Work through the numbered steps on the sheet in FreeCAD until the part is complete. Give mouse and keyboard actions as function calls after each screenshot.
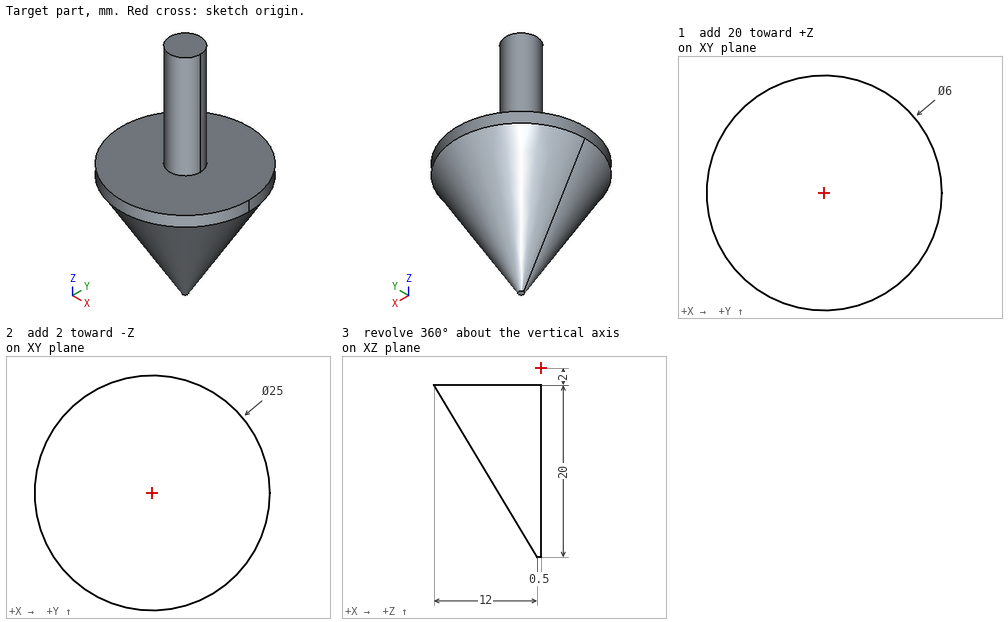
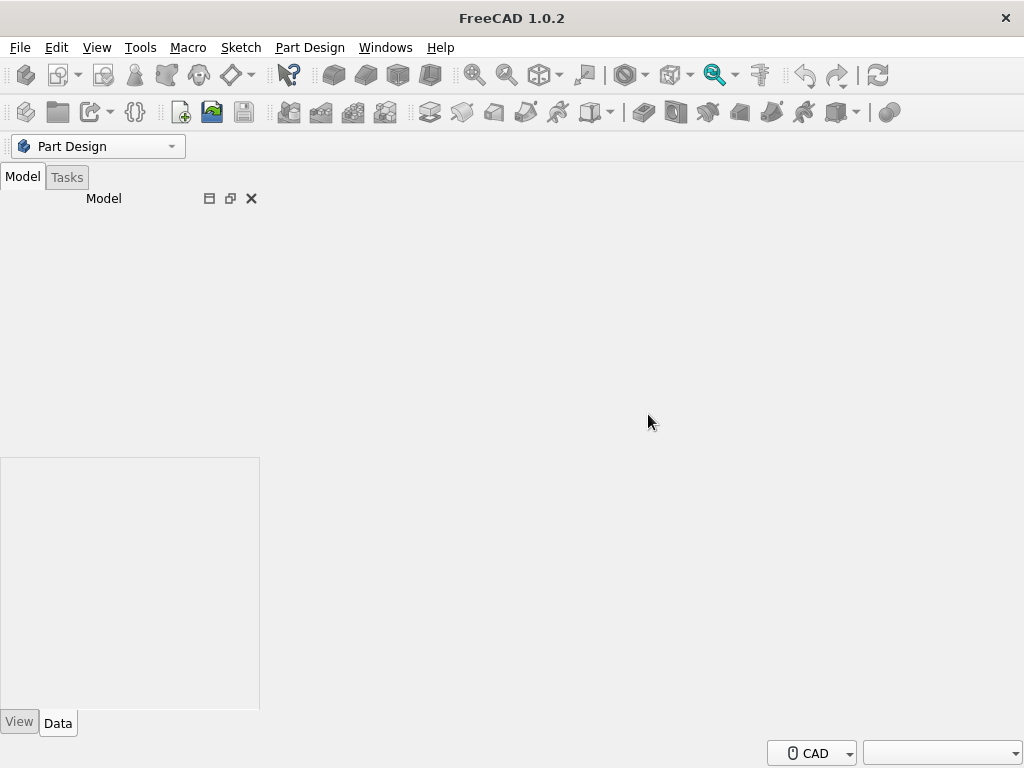
click(180, 112)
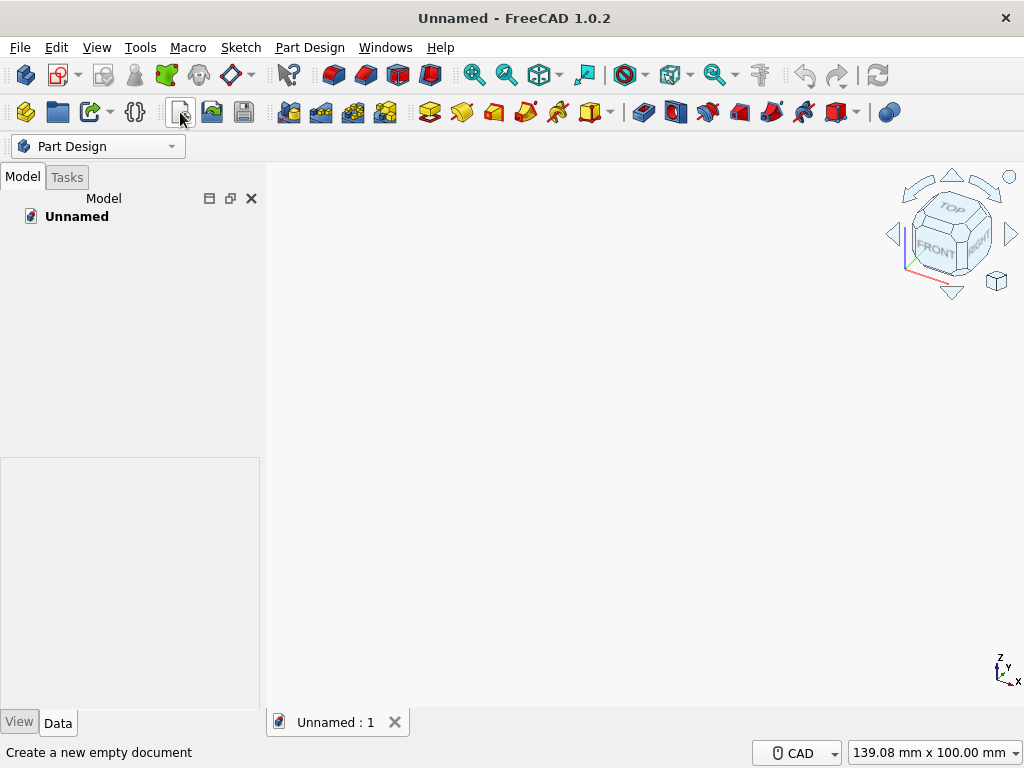
click(58, 76)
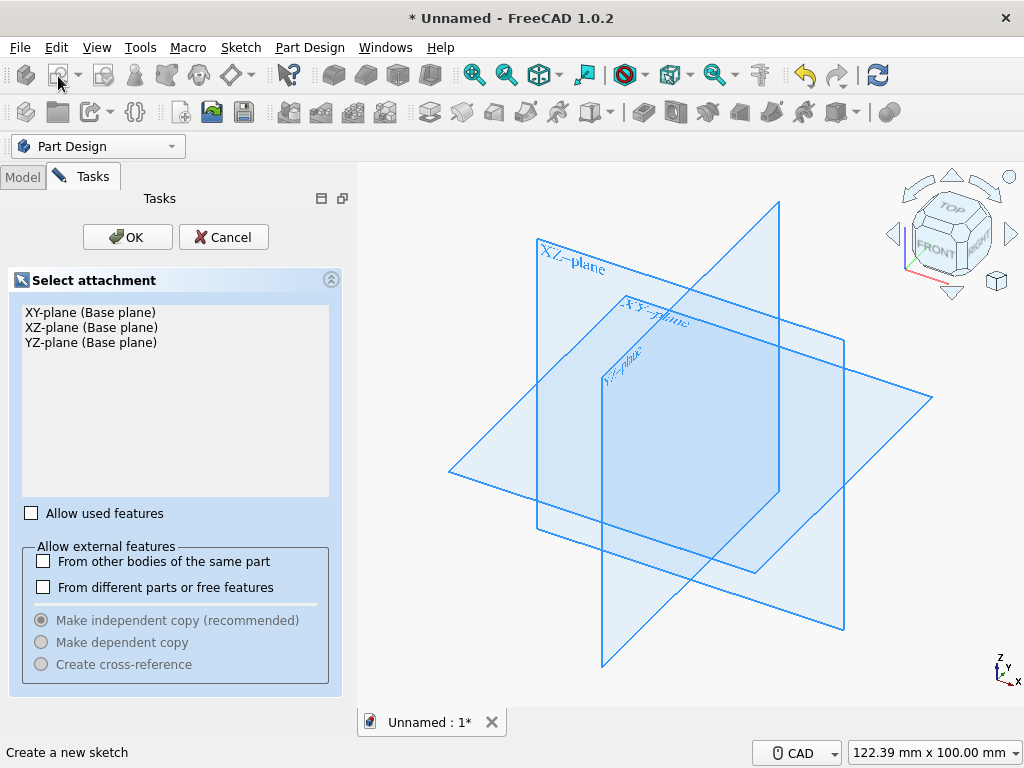
click(82, 312)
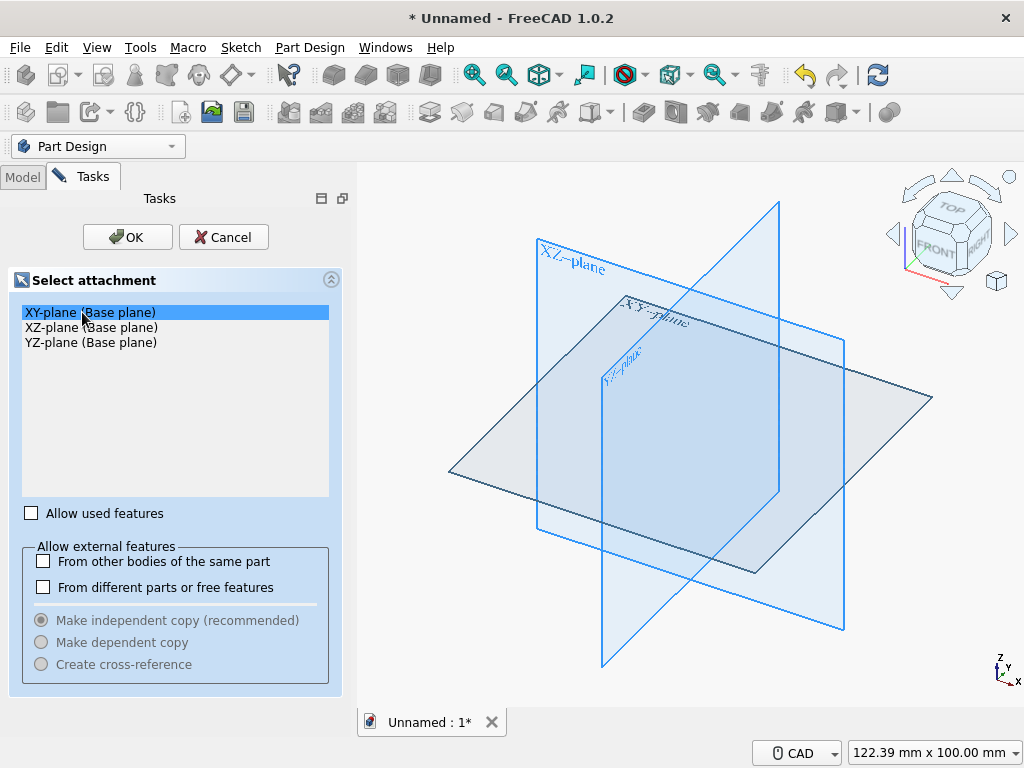
click(128, 237)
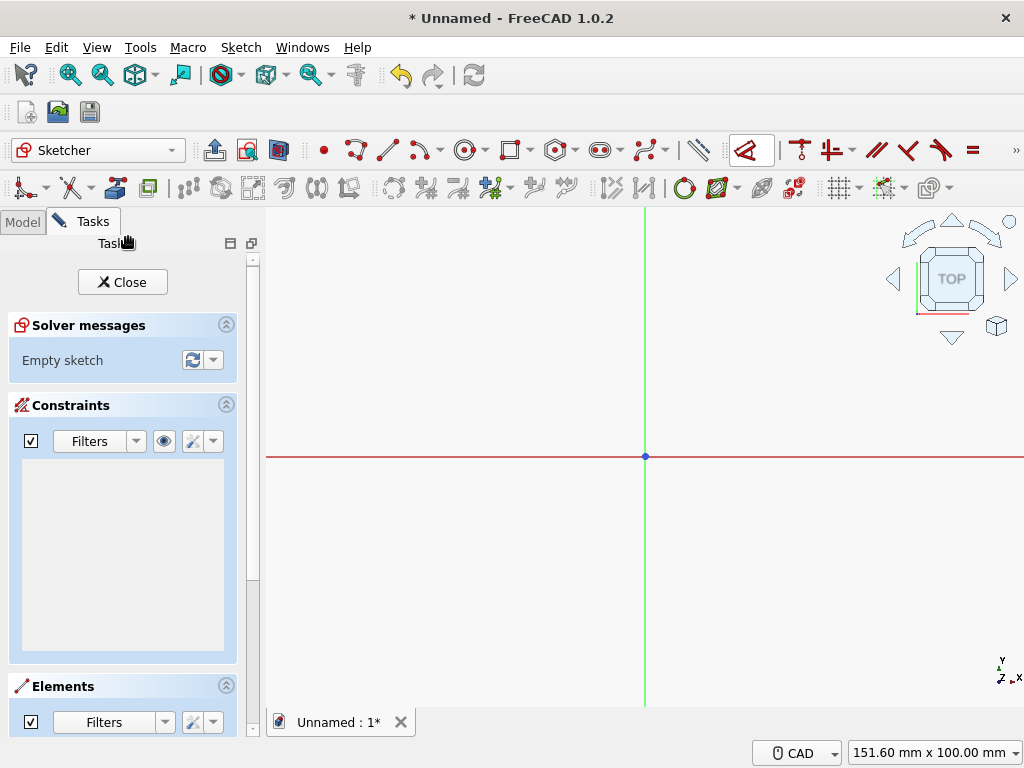
scroll(652, 457, up, 12)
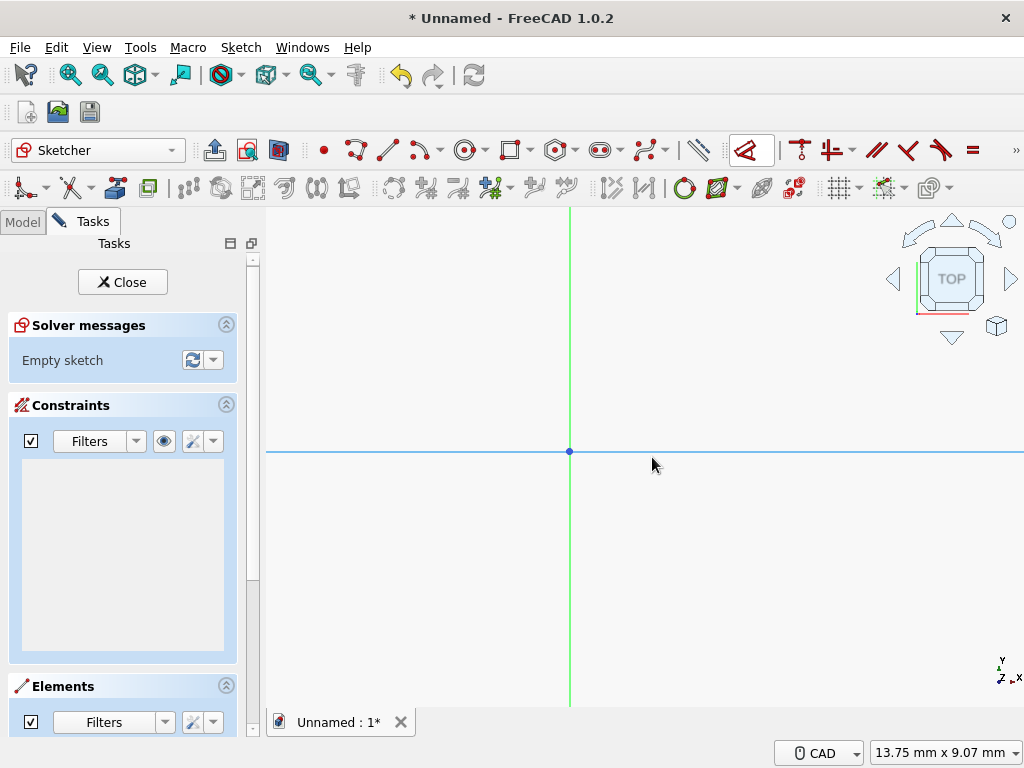
click(466, 150)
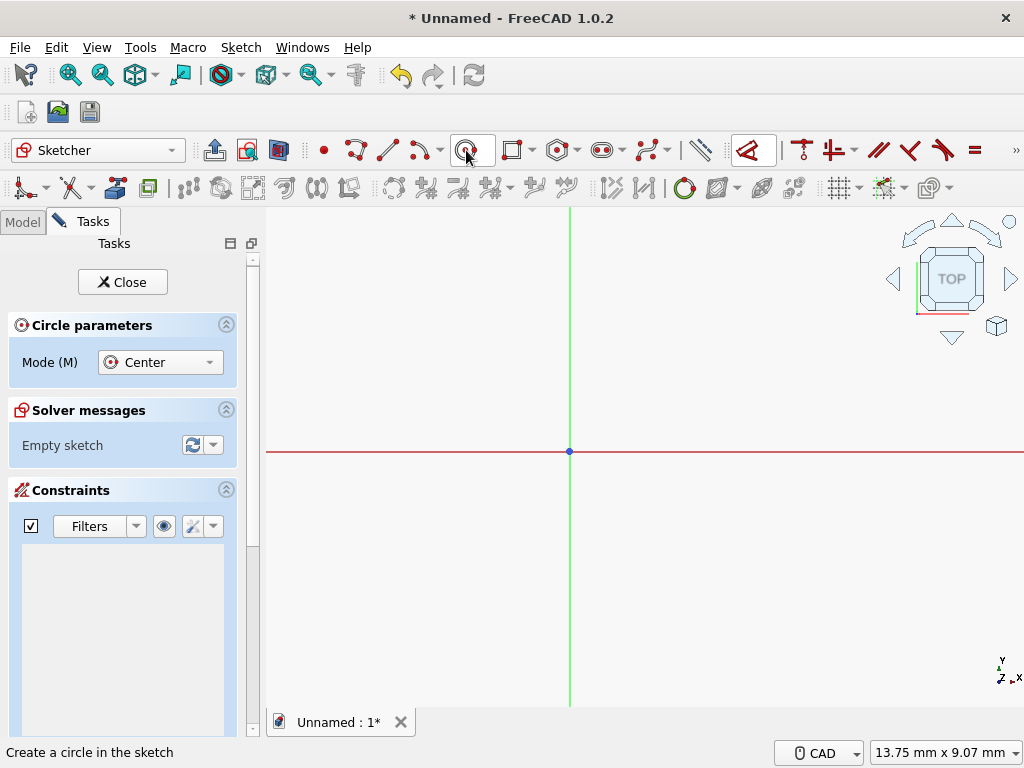
click(570, 452)
click(687, 335)
key(Escape)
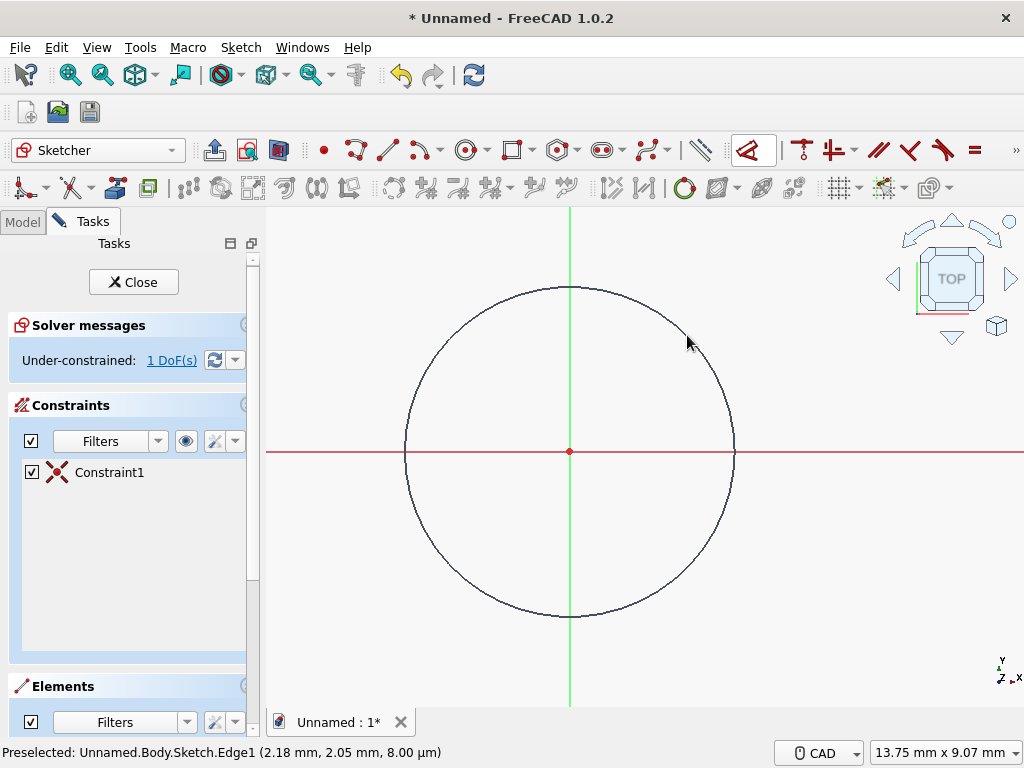
click(748, 150)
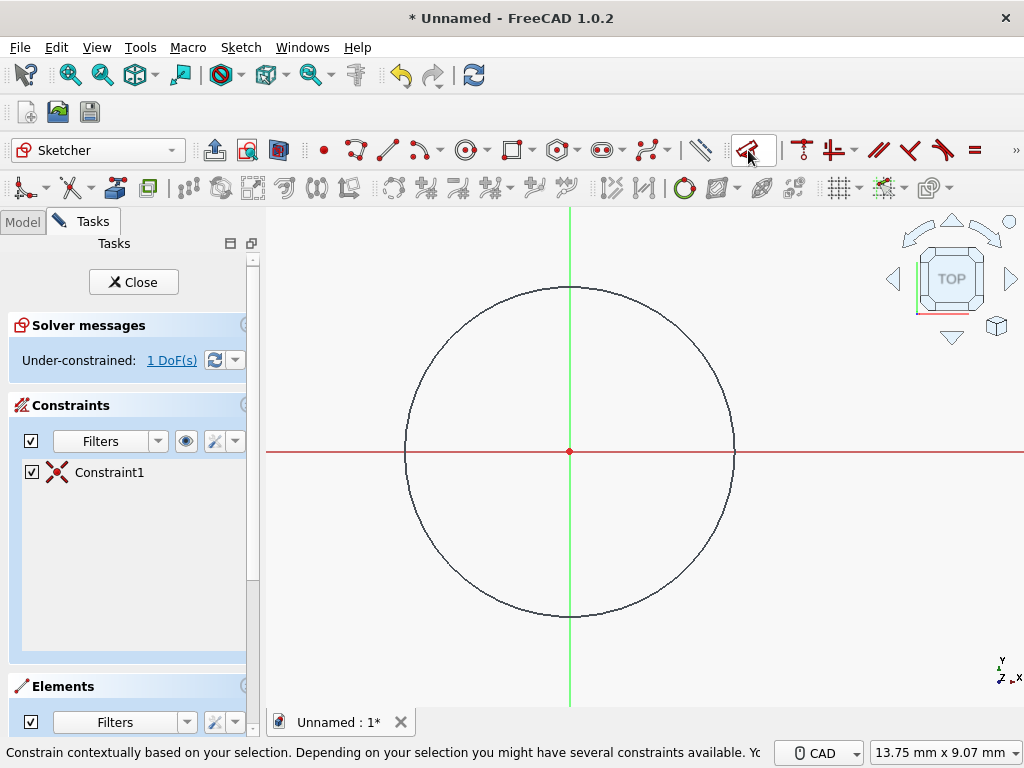
click(686, 335)
click(709, 312)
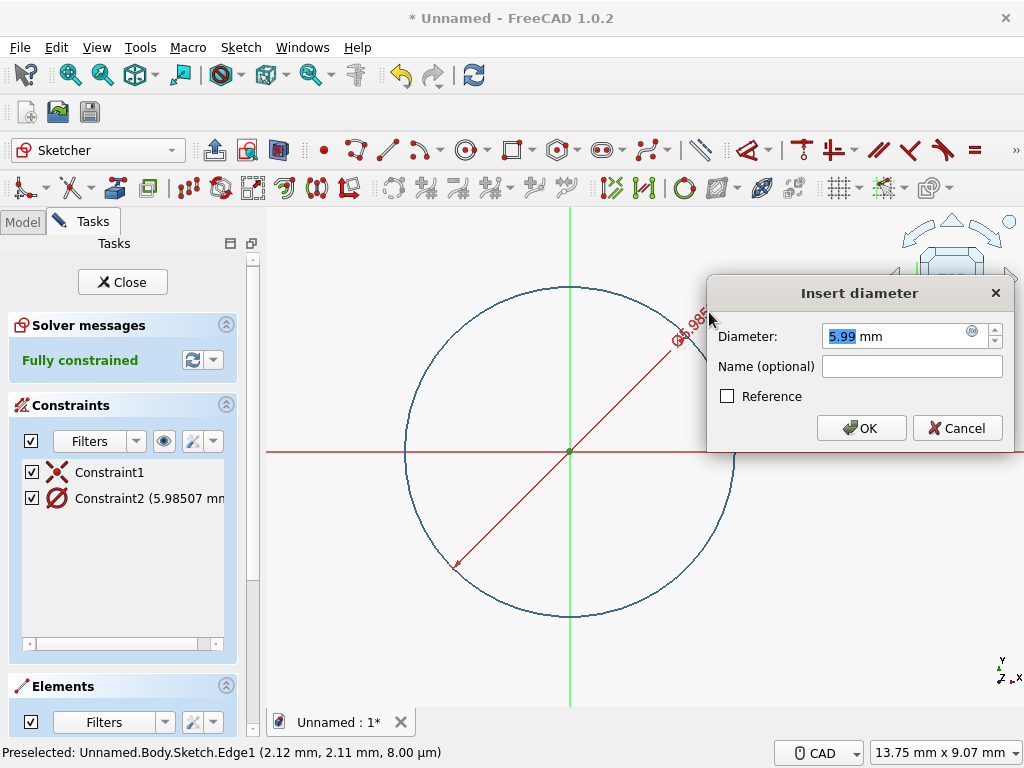
text(6)
key(Return)
key(Escape)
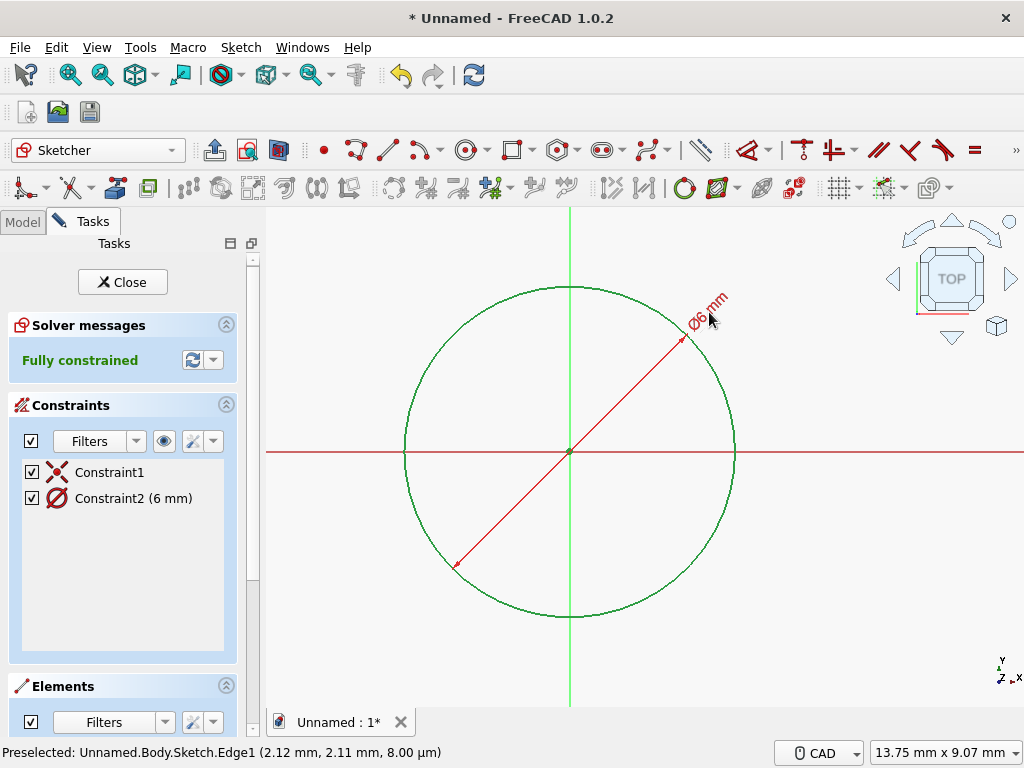
click(123, 282)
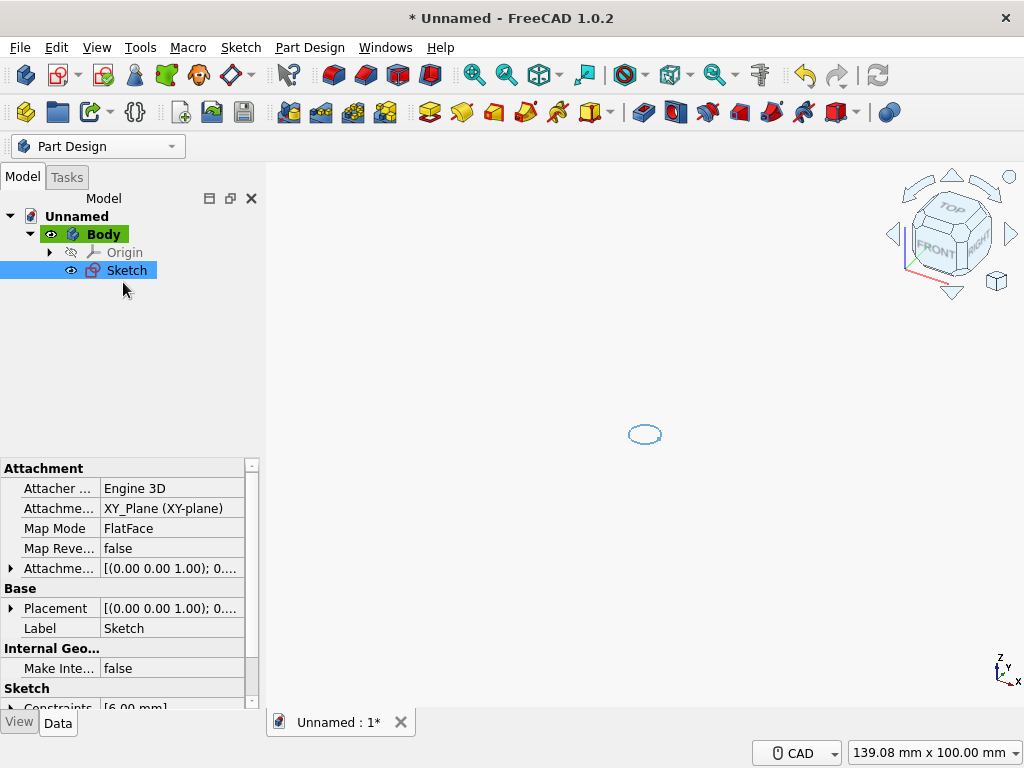
click(430, 112)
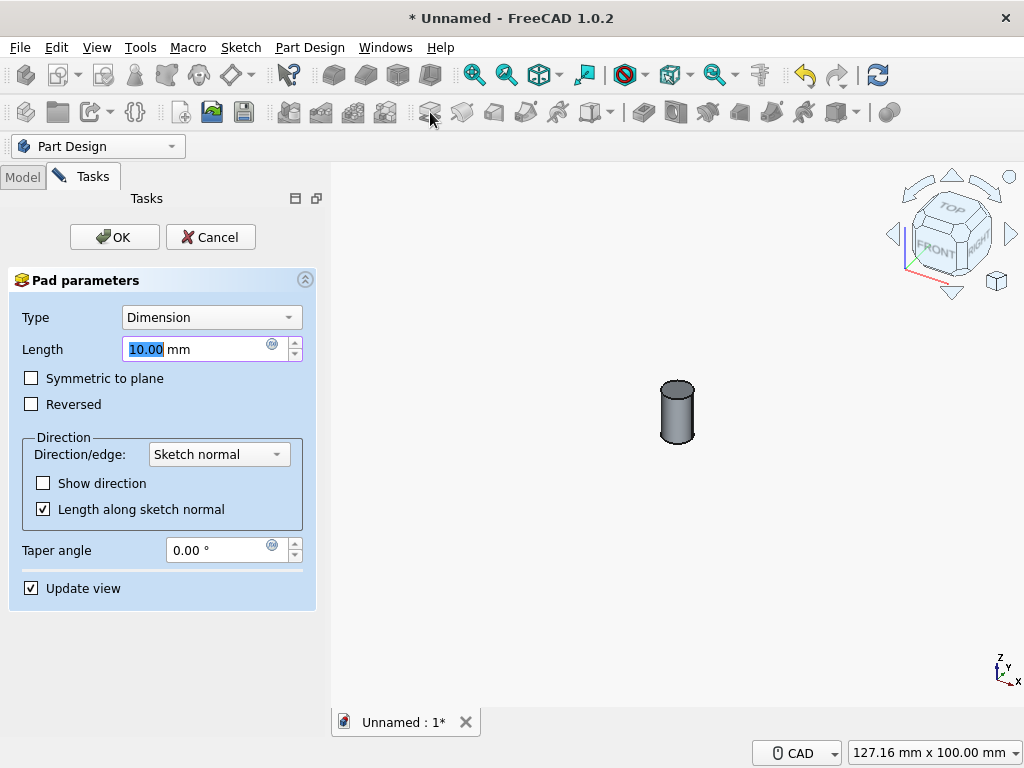
text(20)
key(Tab)